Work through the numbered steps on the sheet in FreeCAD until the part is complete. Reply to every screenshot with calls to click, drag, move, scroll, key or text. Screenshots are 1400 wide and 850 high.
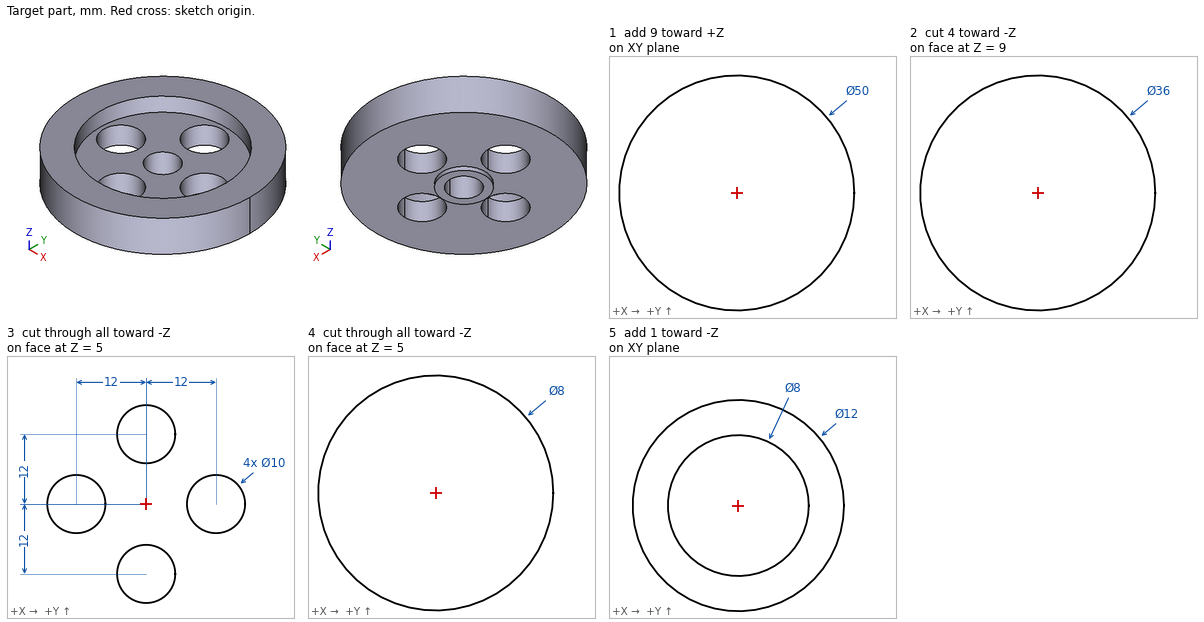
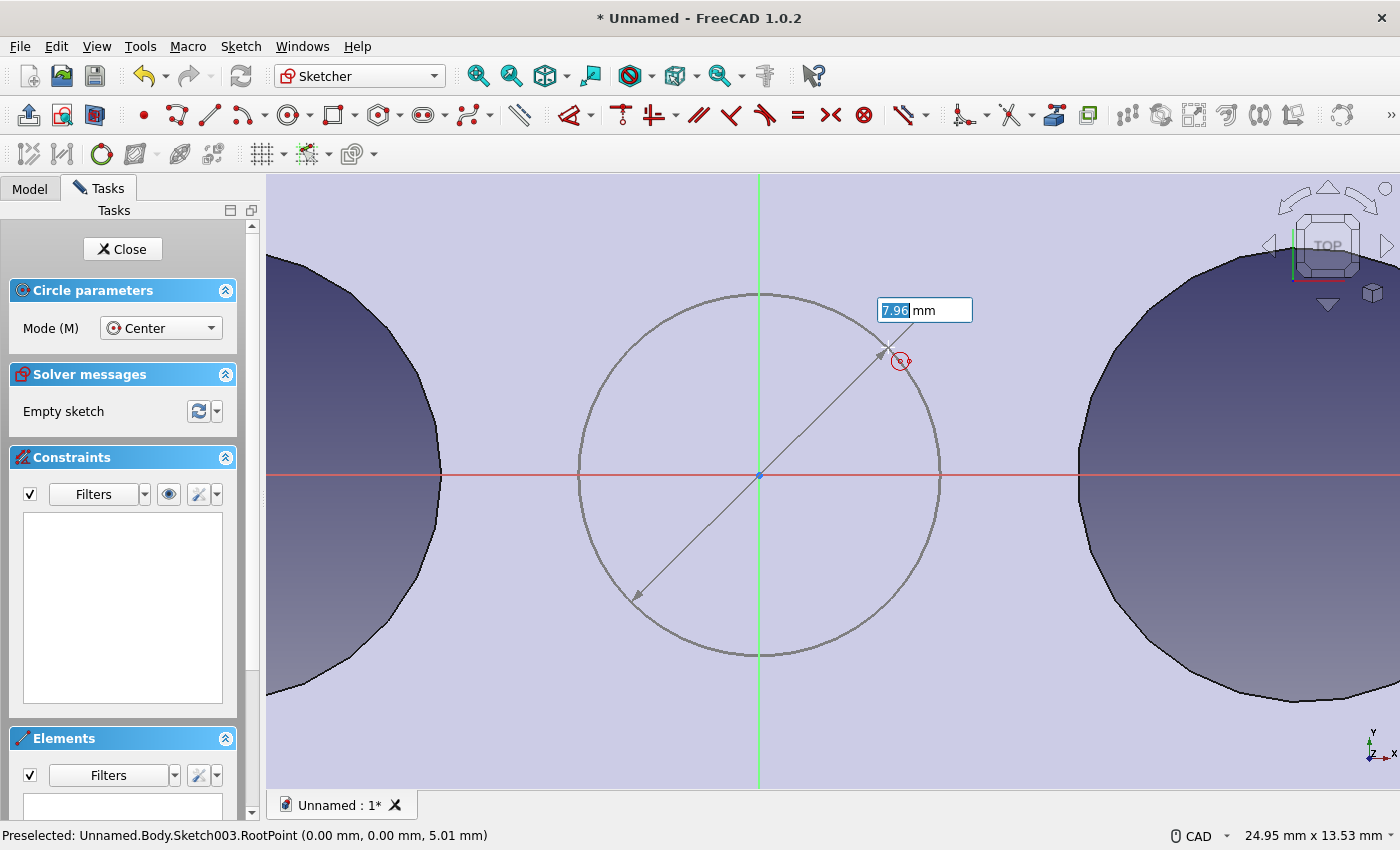
text(8)
key(Return)
key(Escape)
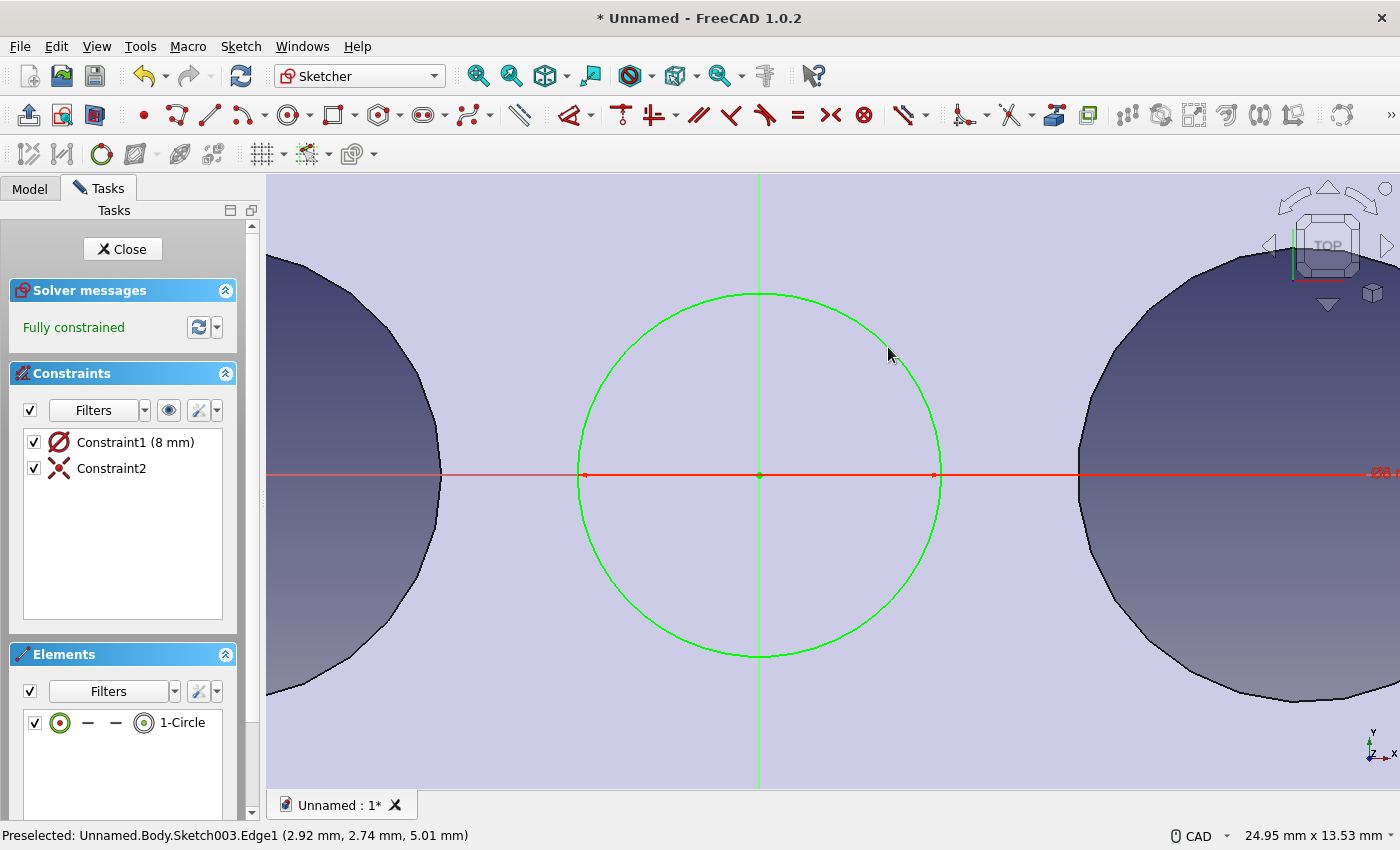
click(123, 249)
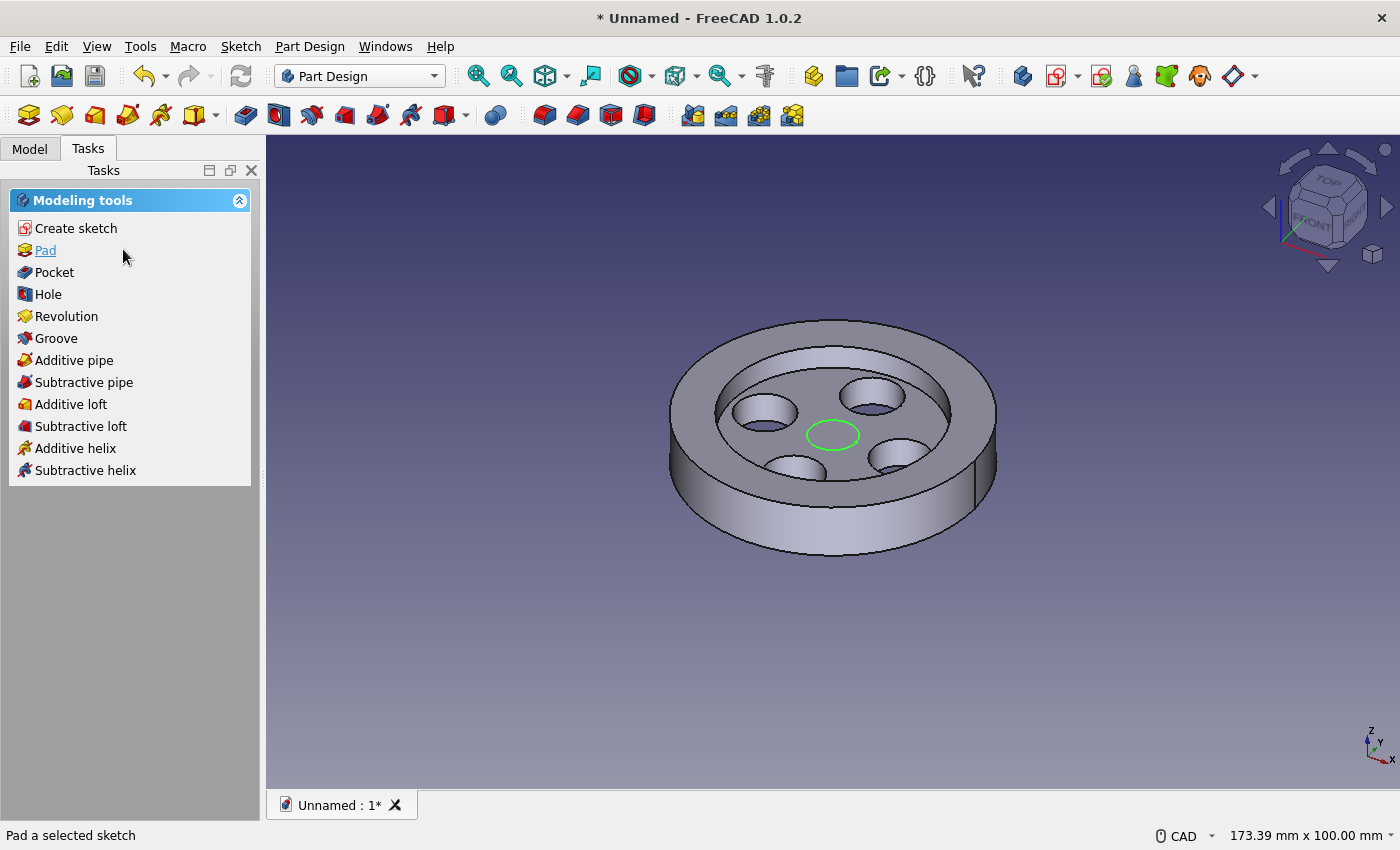
click(246, 116)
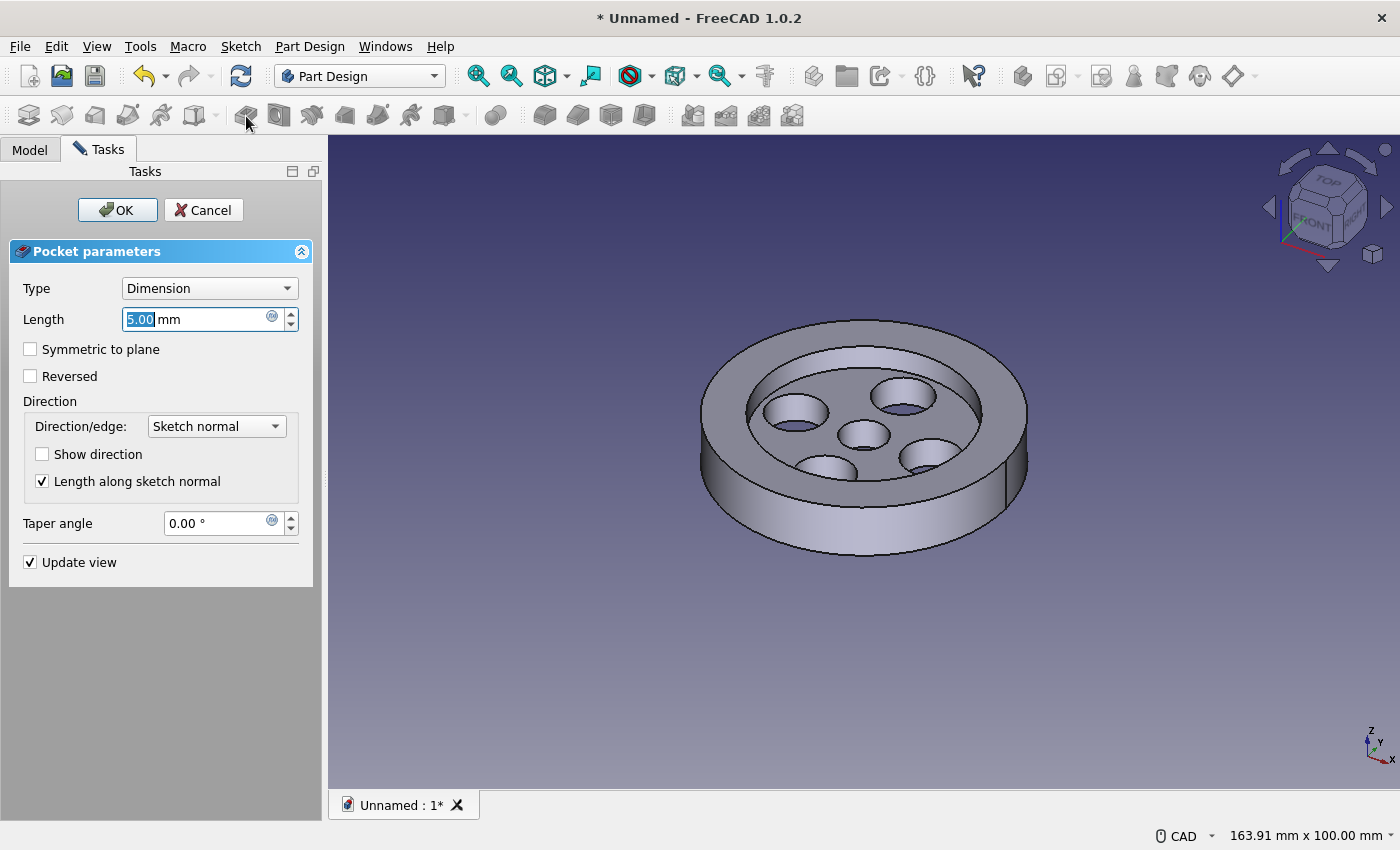
click(210, 288)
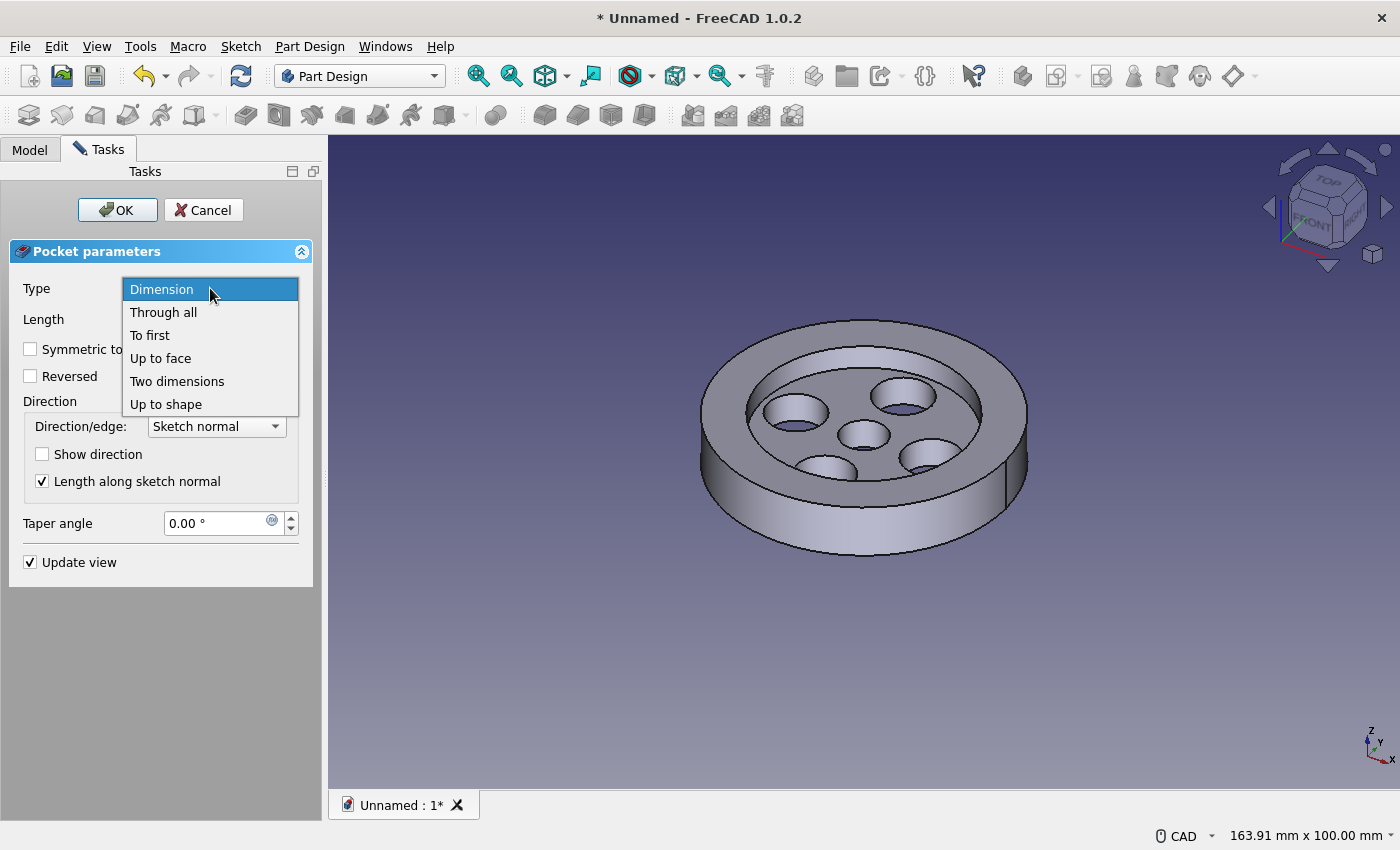
click(208, 312)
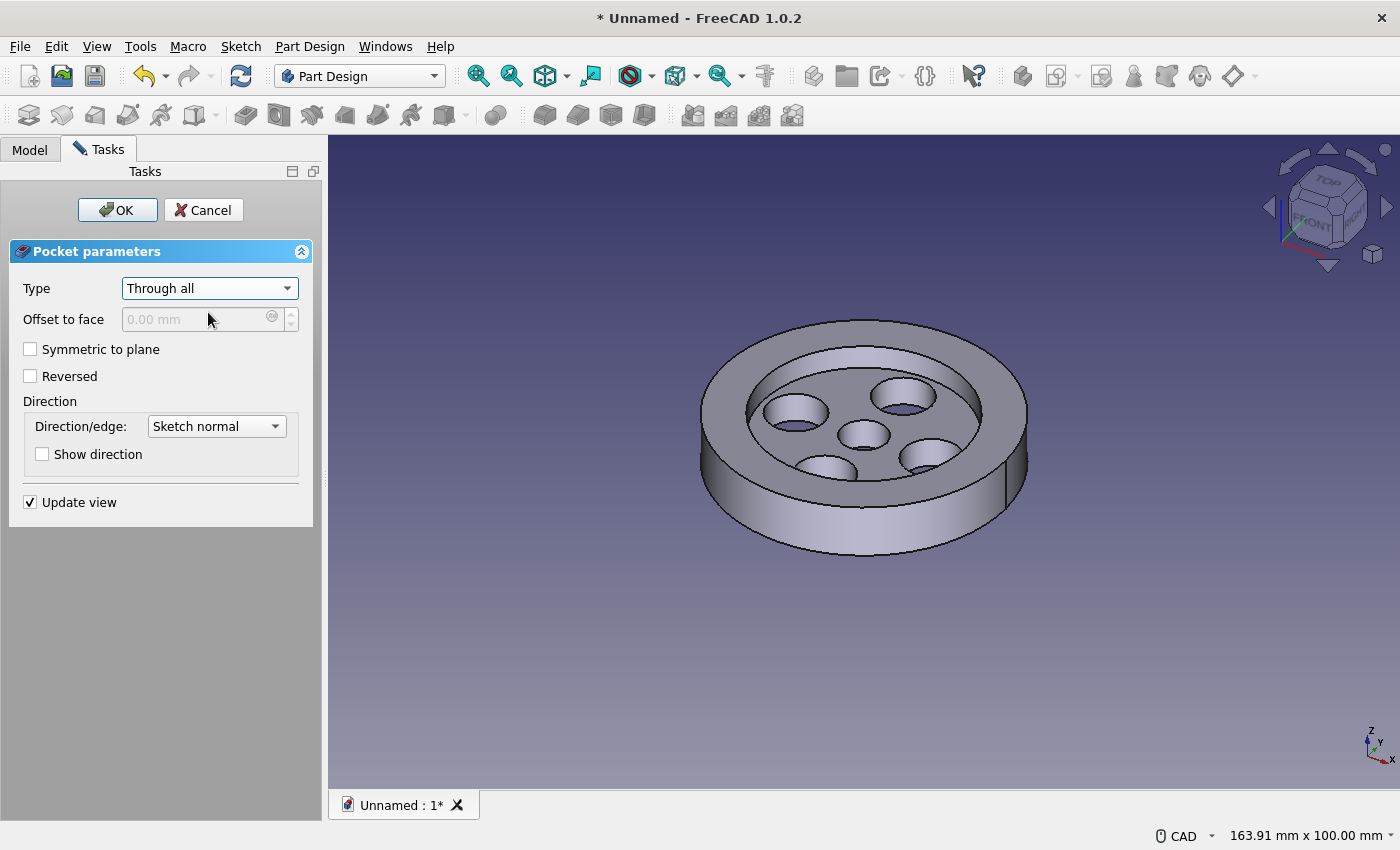
click(118, 210)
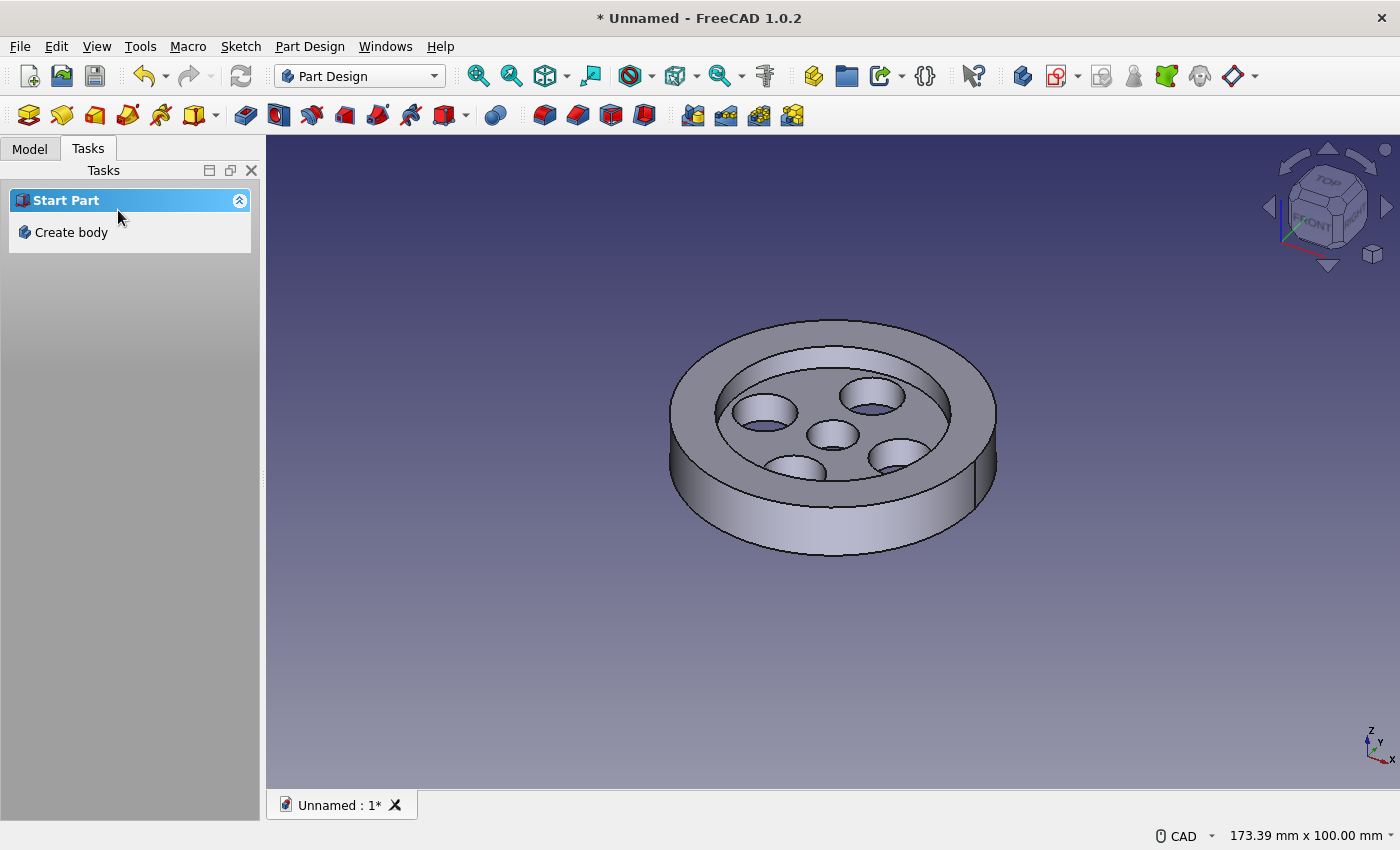
click(1056, 76)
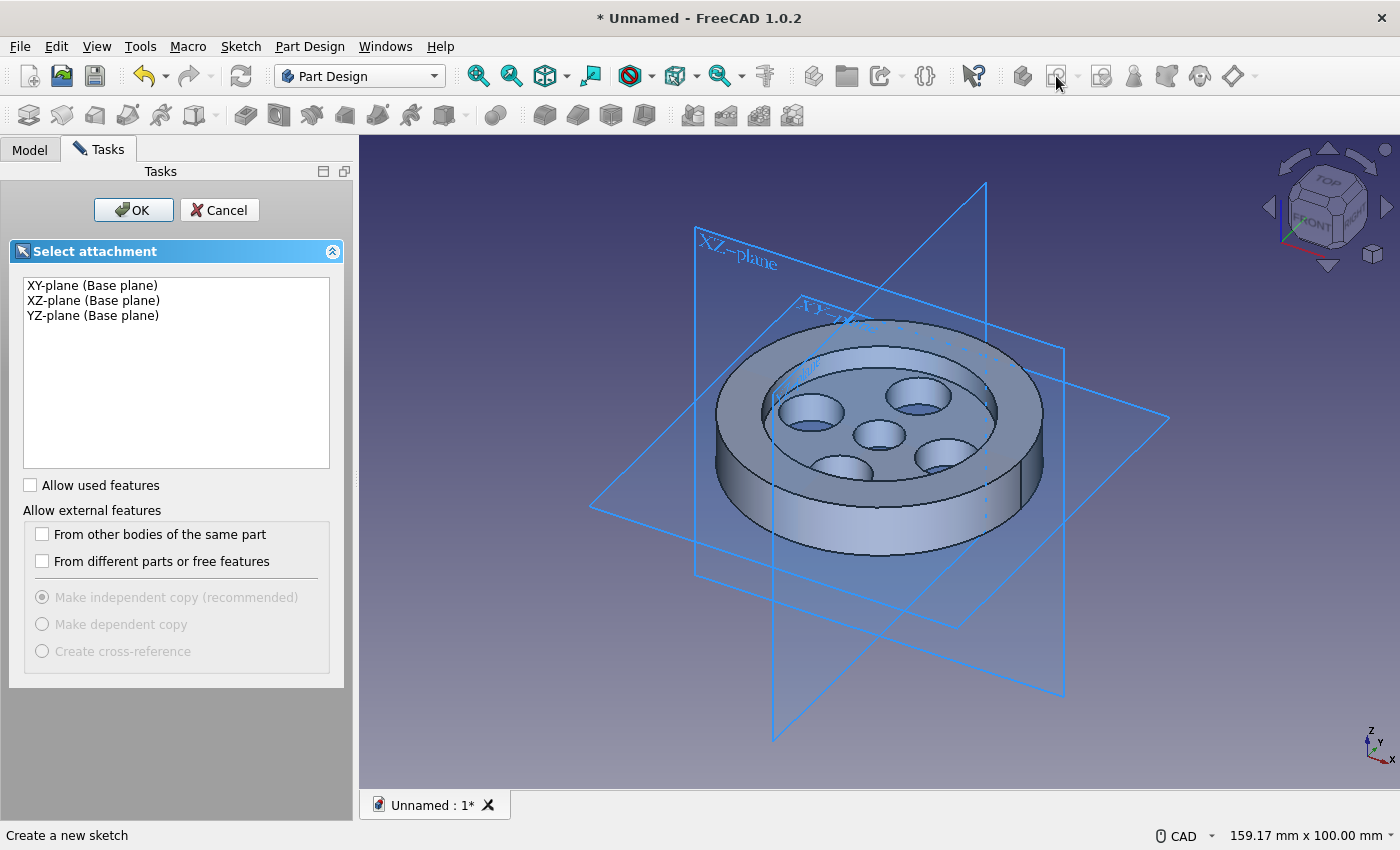
click(84, 286)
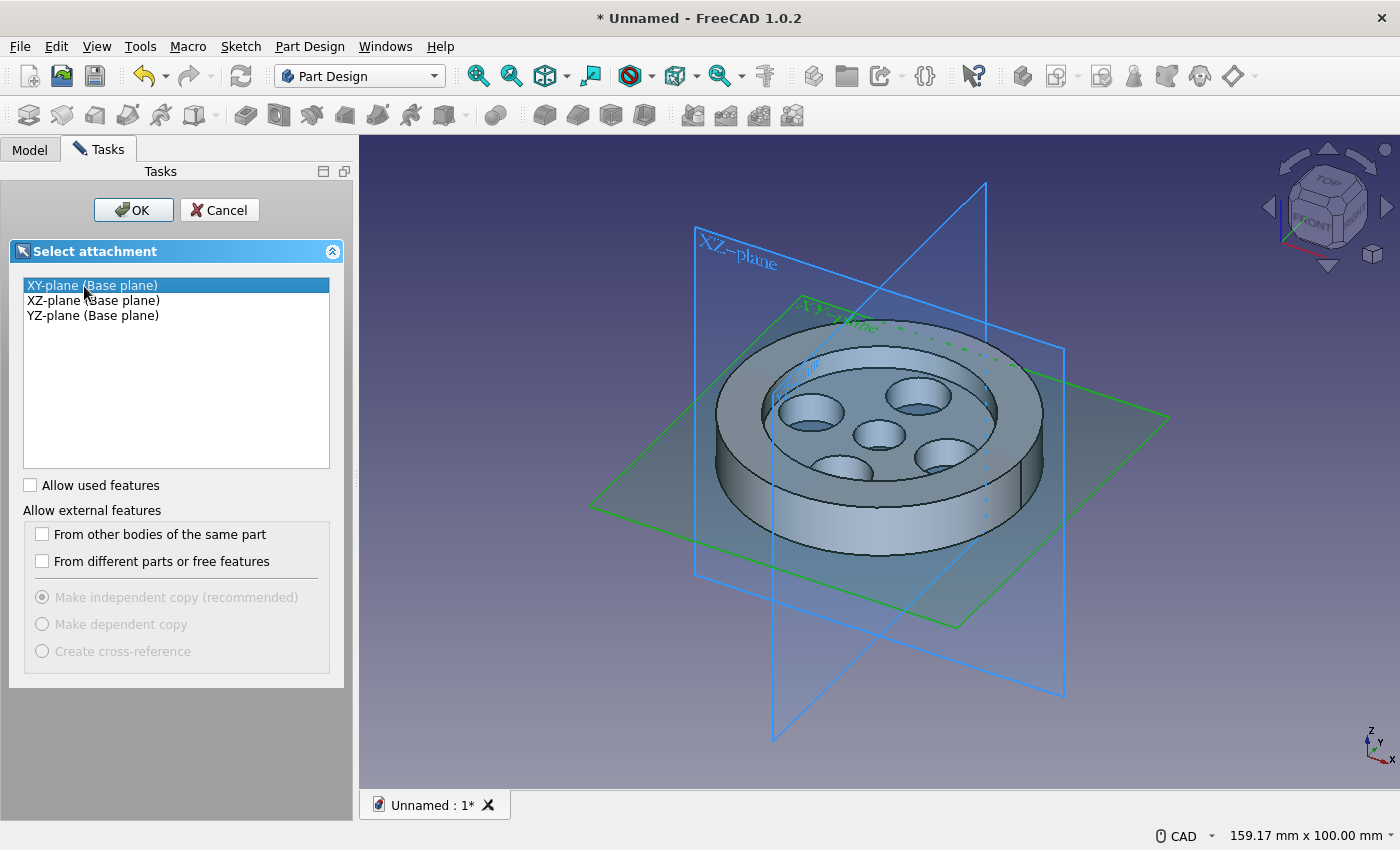
click(134, 210)